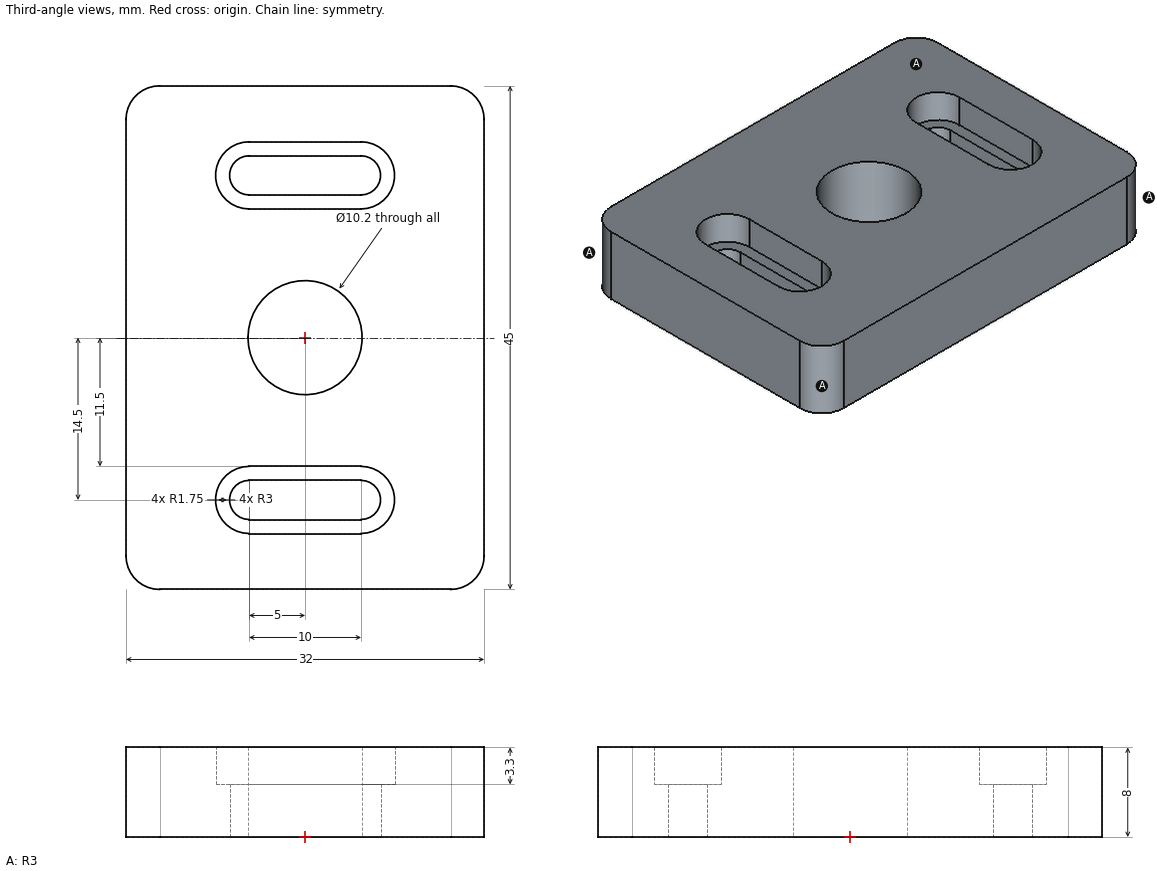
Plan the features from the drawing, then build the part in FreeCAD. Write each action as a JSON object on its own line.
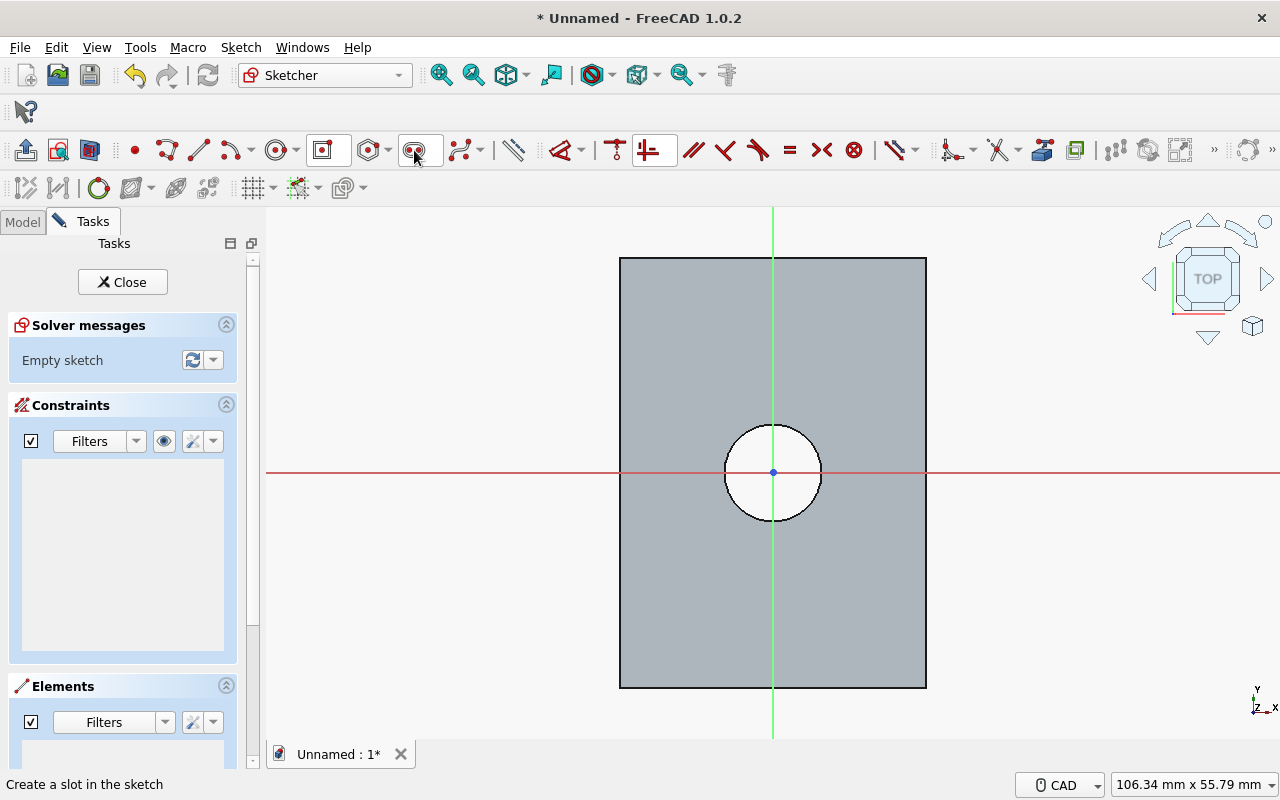
{"action": "scroll", "coordinate": [725, 611], "scroll_direction": "up", "scroll_amount": 2}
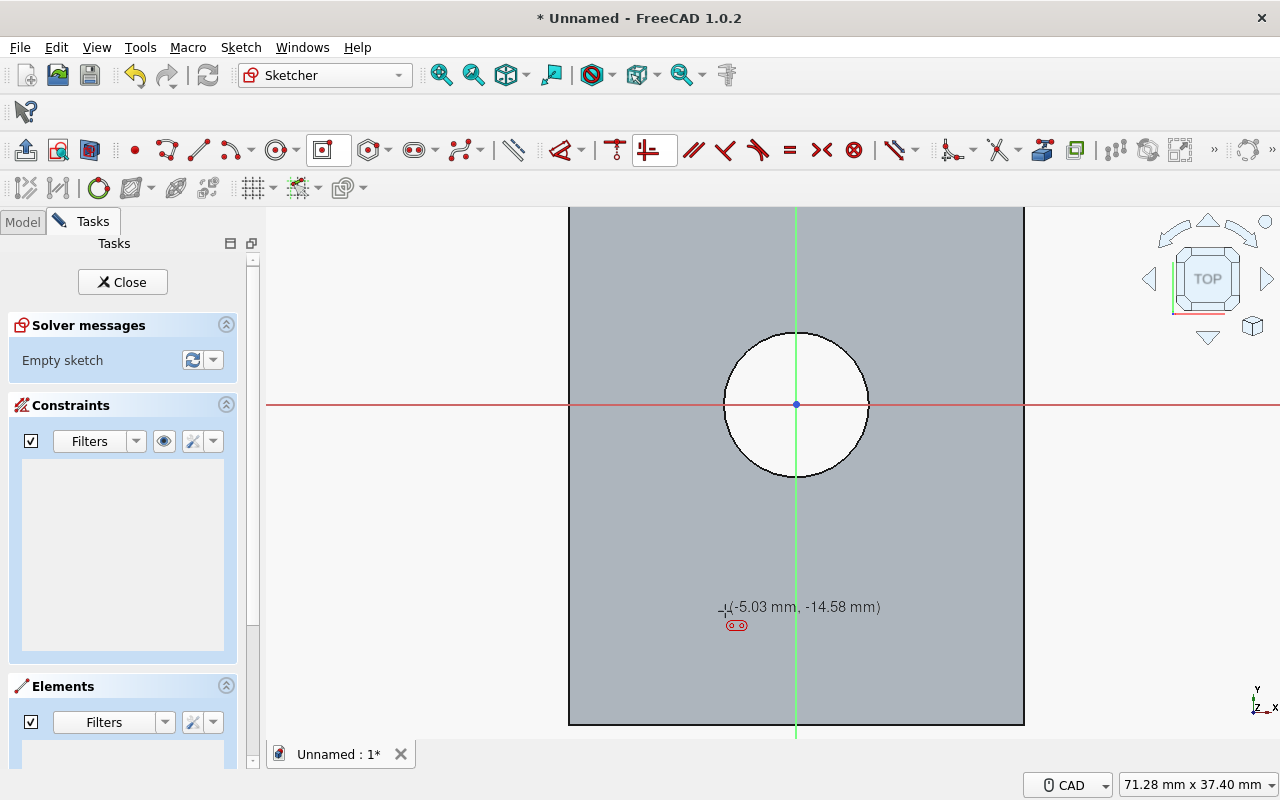
{"action": "left_click", "coordinate": [725, 611]}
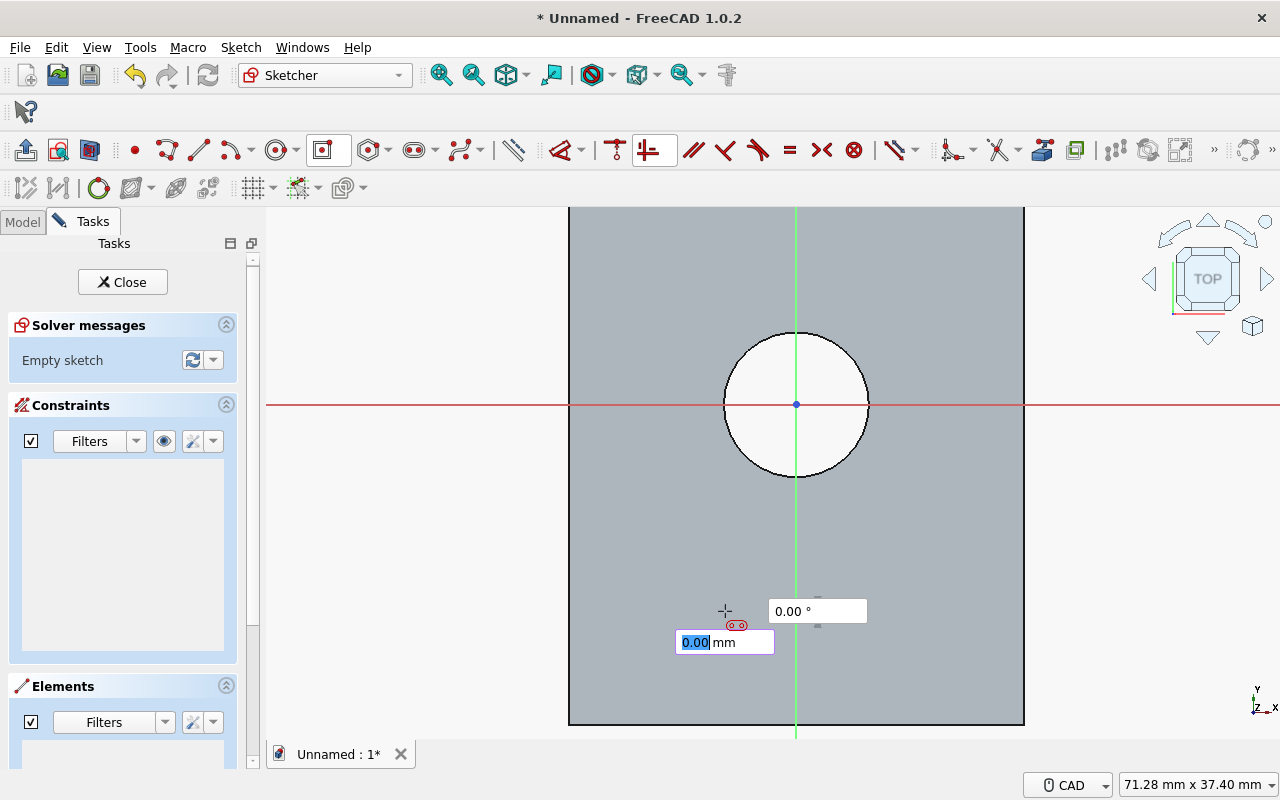
{"action": "left_click", "coordinate": [868, 611]}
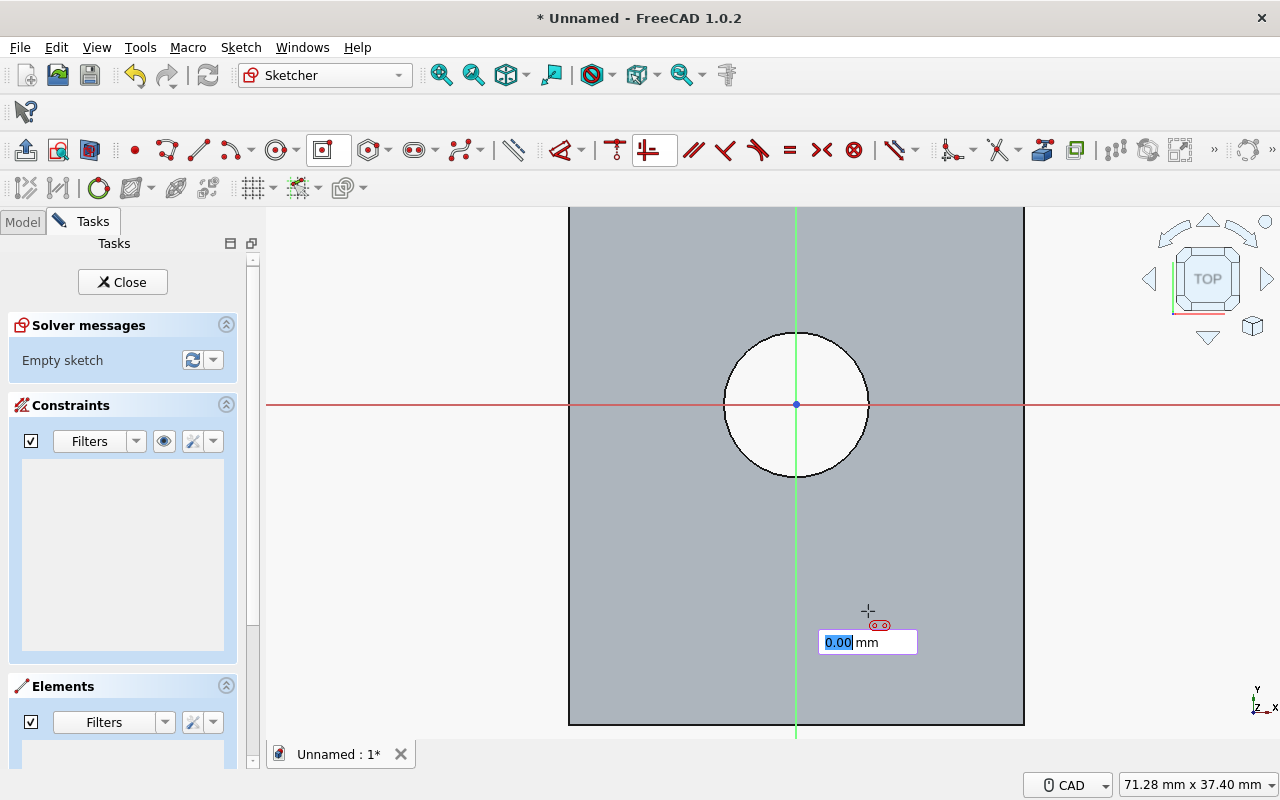
{"action": "left_click", "coordinate": [818, 586]}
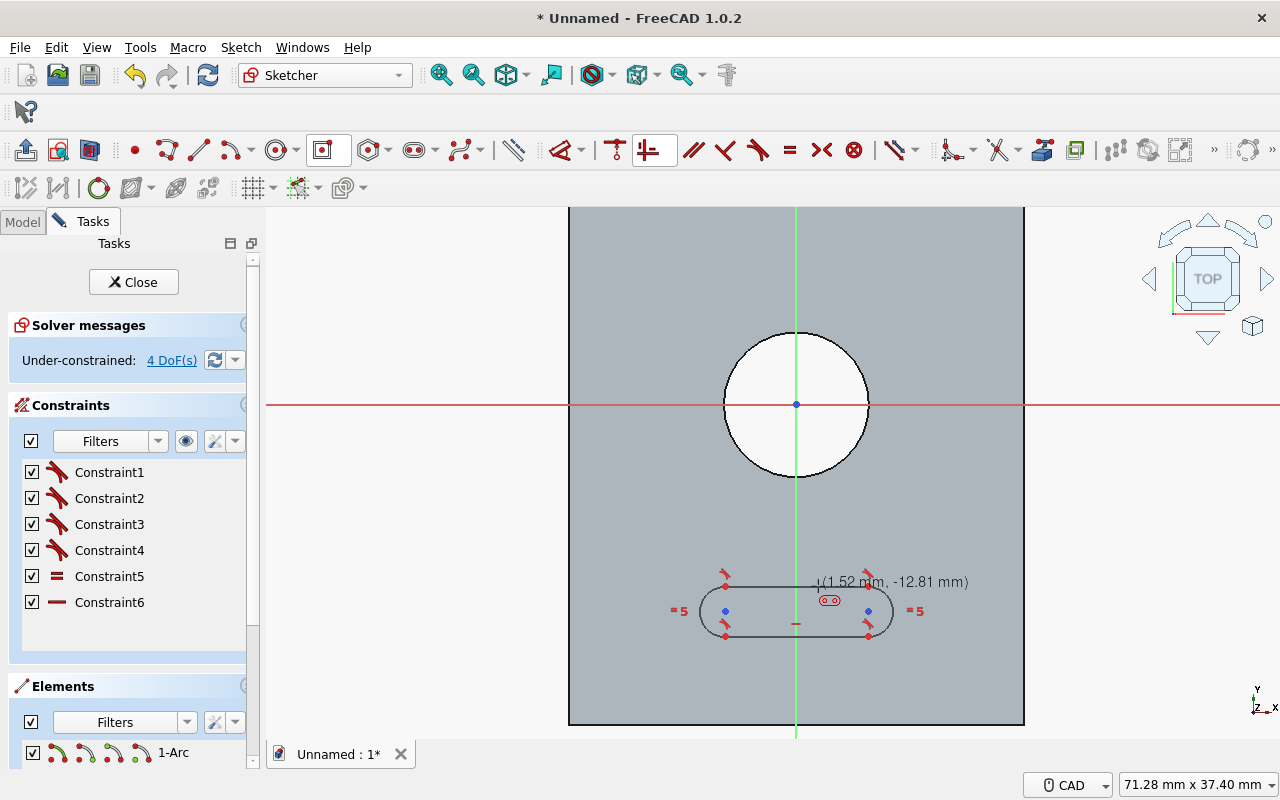
{"action": "scroll", "coordinate": [518, 612], "scroll_direction": "down", "scroll_amount": 2}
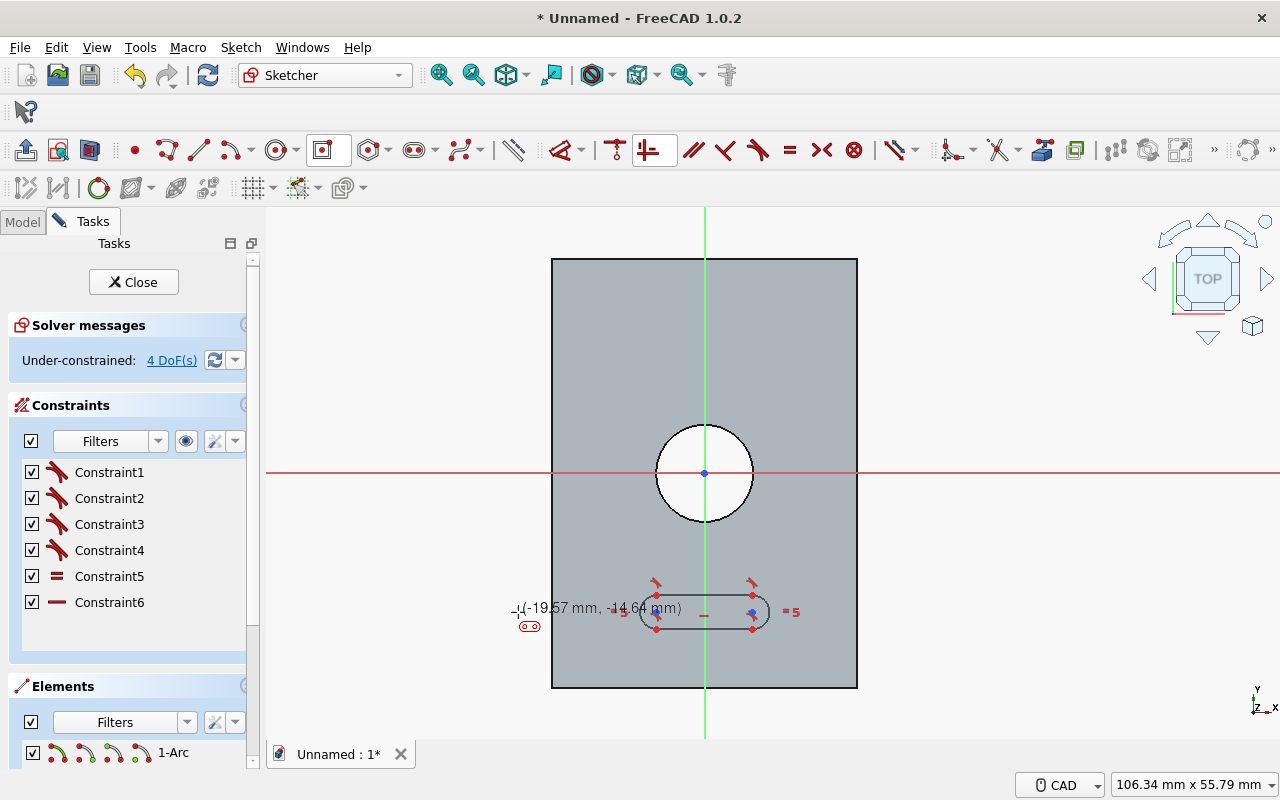
{"action": "scroll", "coordinate": [657, 335], "scroll_direction": "up", "scroll_amount": 2}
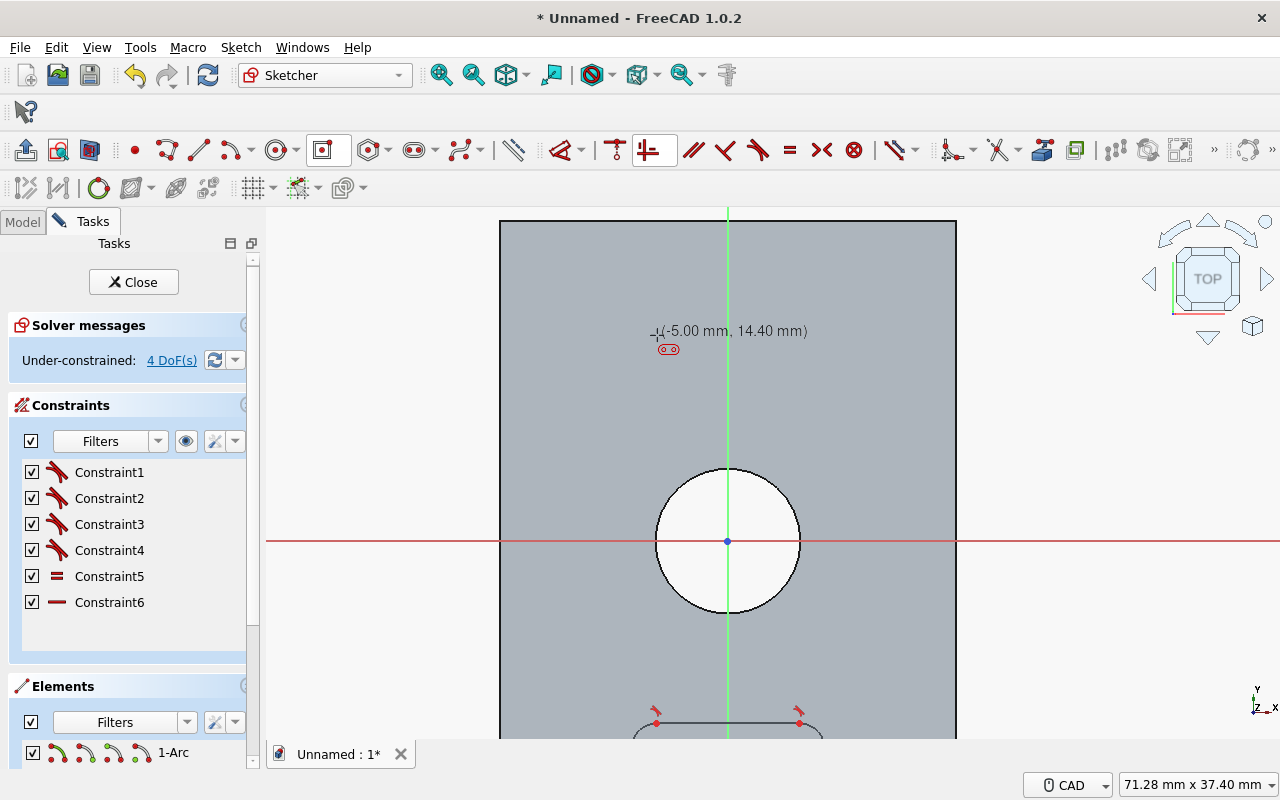
{"action": "left_click", "coordinate": [657, 335]}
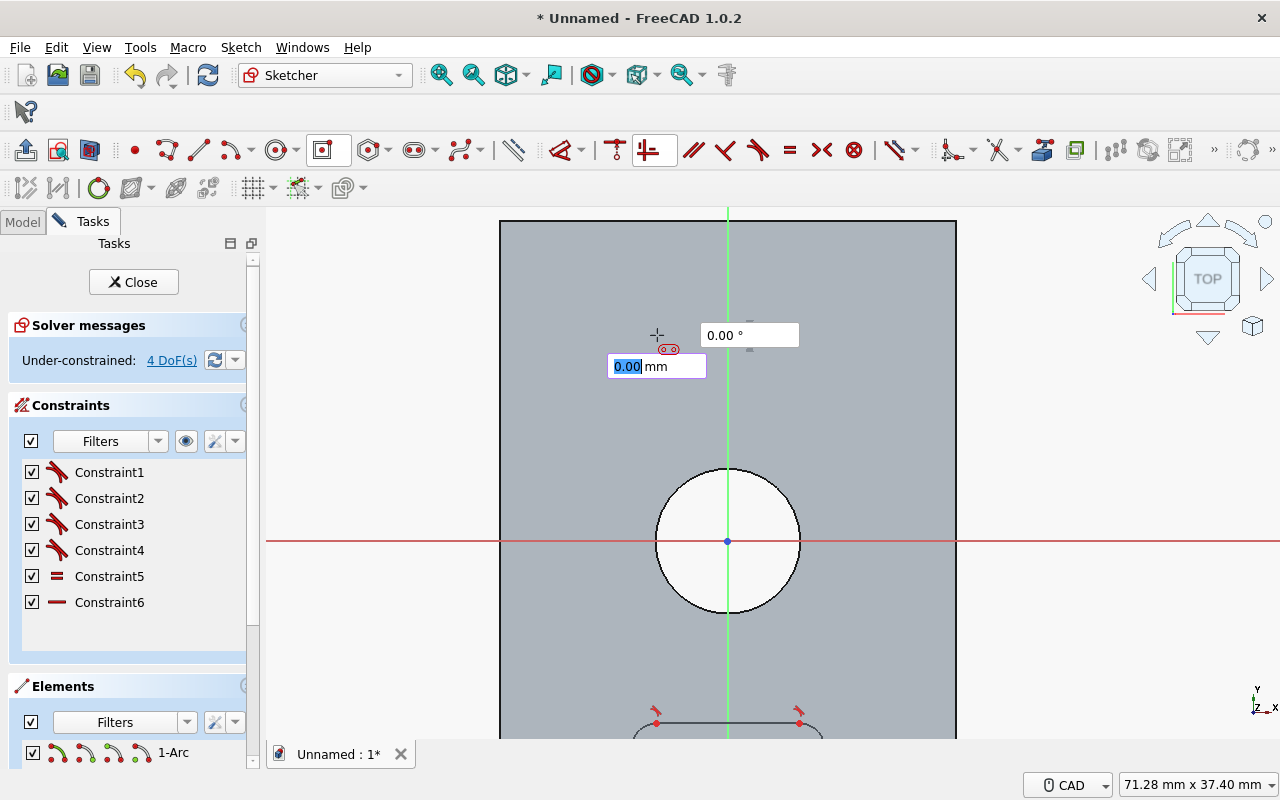
{"action": "left_click", "coordinate": [799, 335]}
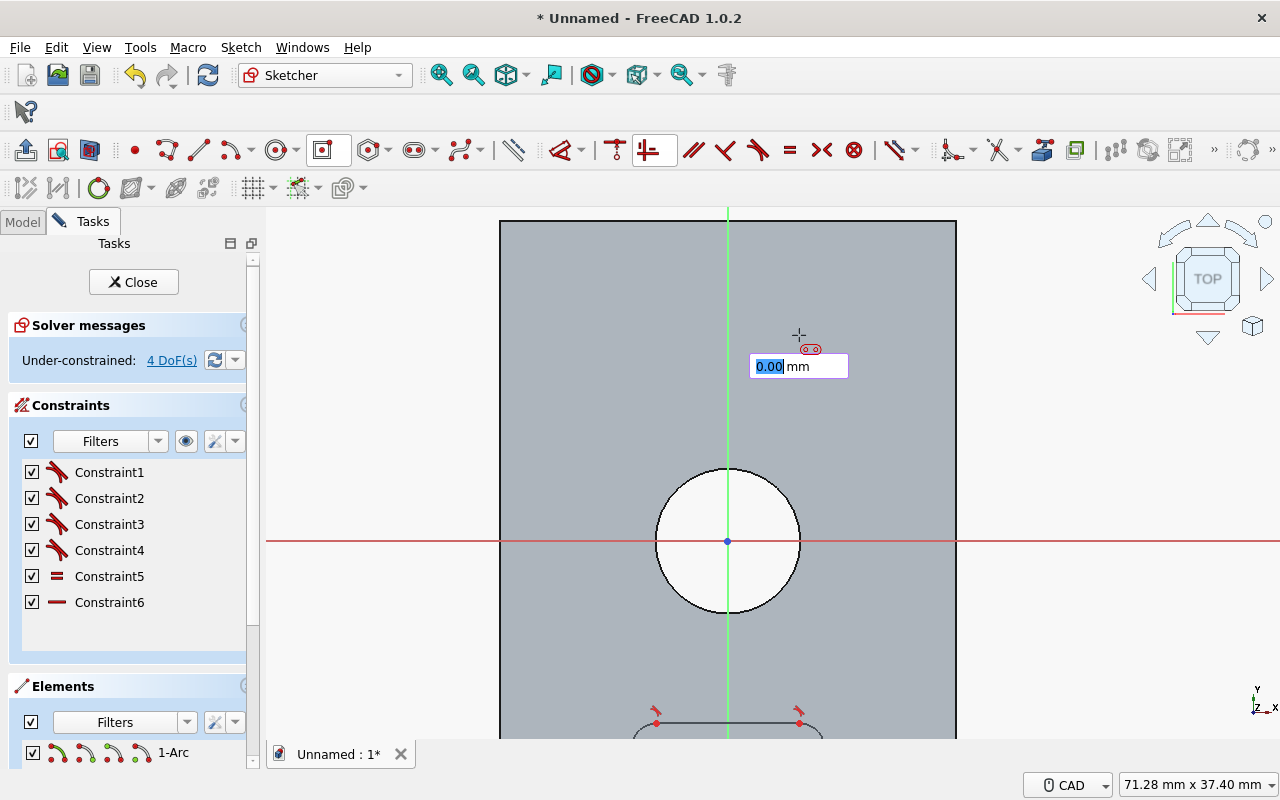
{"action": "left_click", "coordinate": [749, 310]}
{"action": "key", "text": "Escape"}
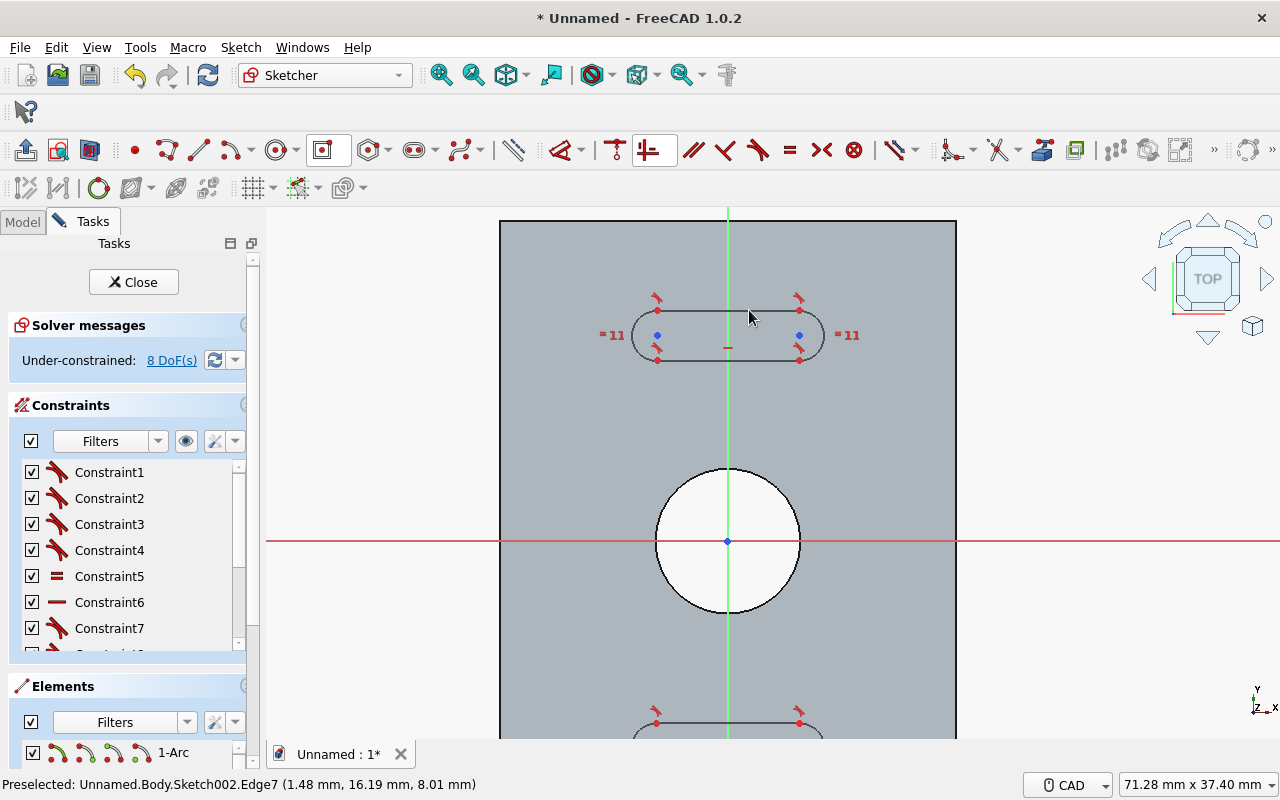
{"action": "scroll", "coordinate": [657, 334], "scroll_direction": "down", "scroll_amount": 2}